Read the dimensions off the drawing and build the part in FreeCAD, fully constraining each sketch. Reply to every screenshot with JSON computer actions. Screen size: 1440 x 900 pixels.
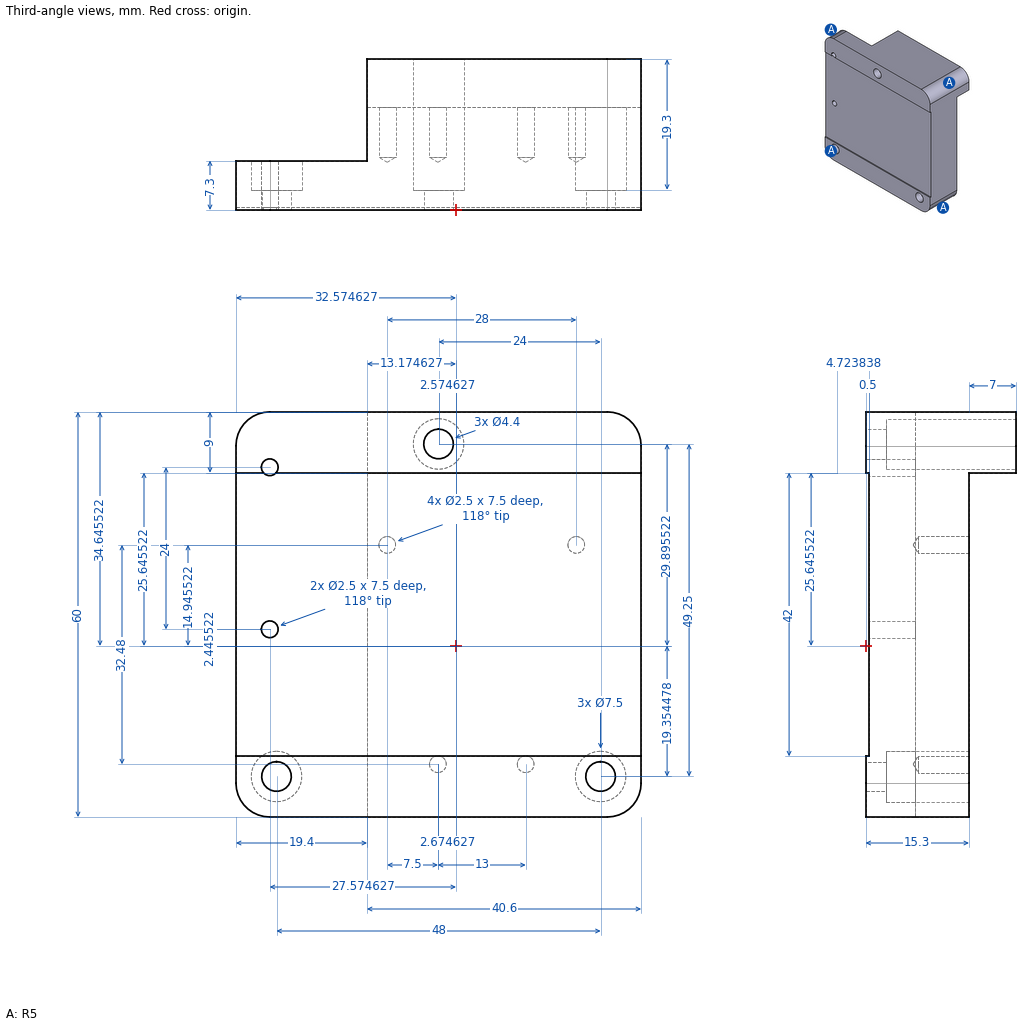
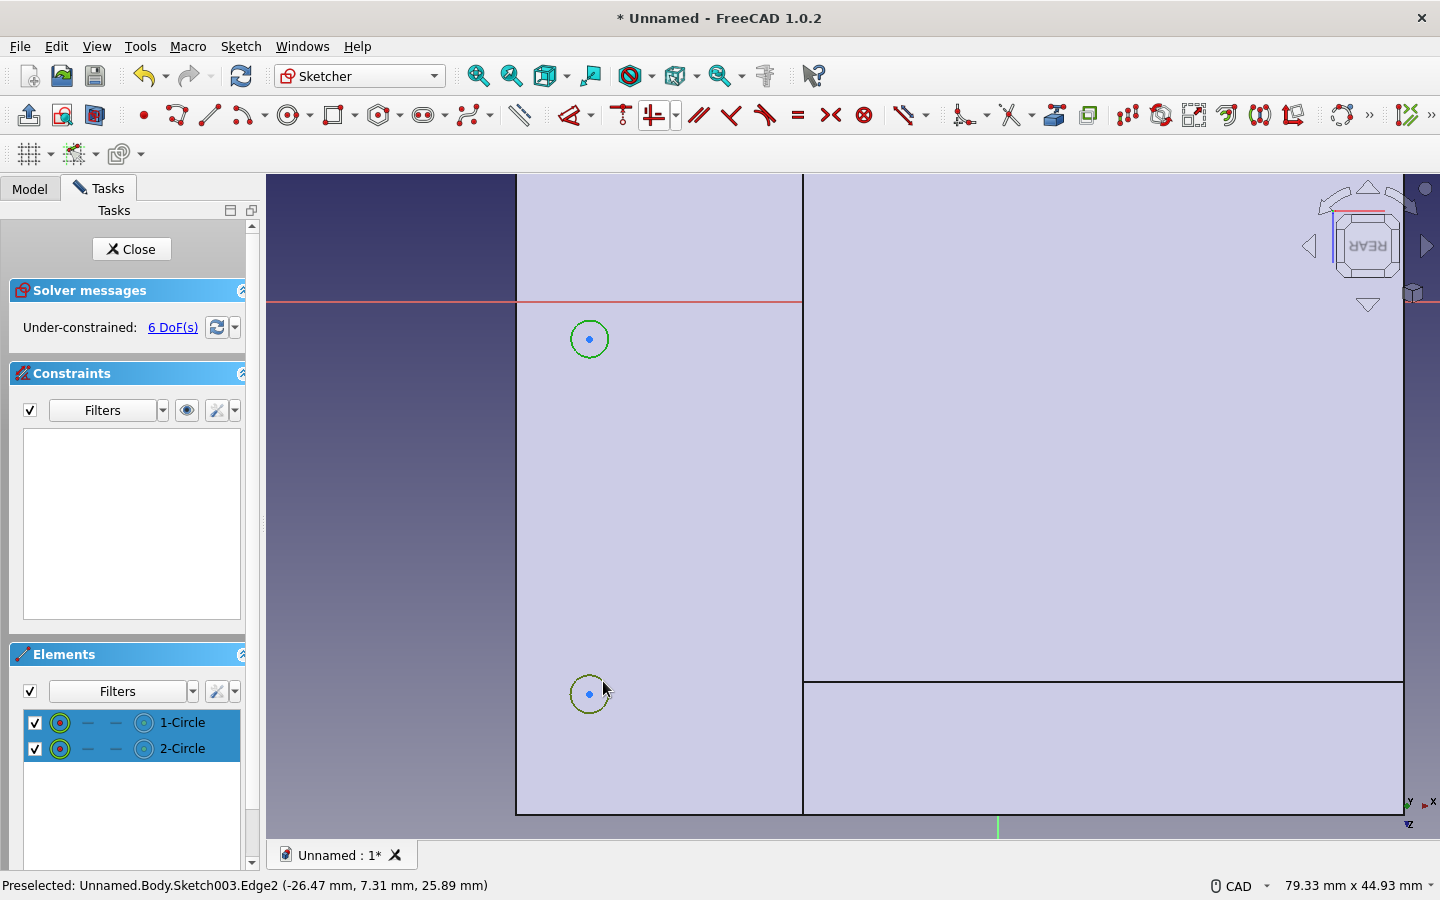
{"action": "key", "text": "e"}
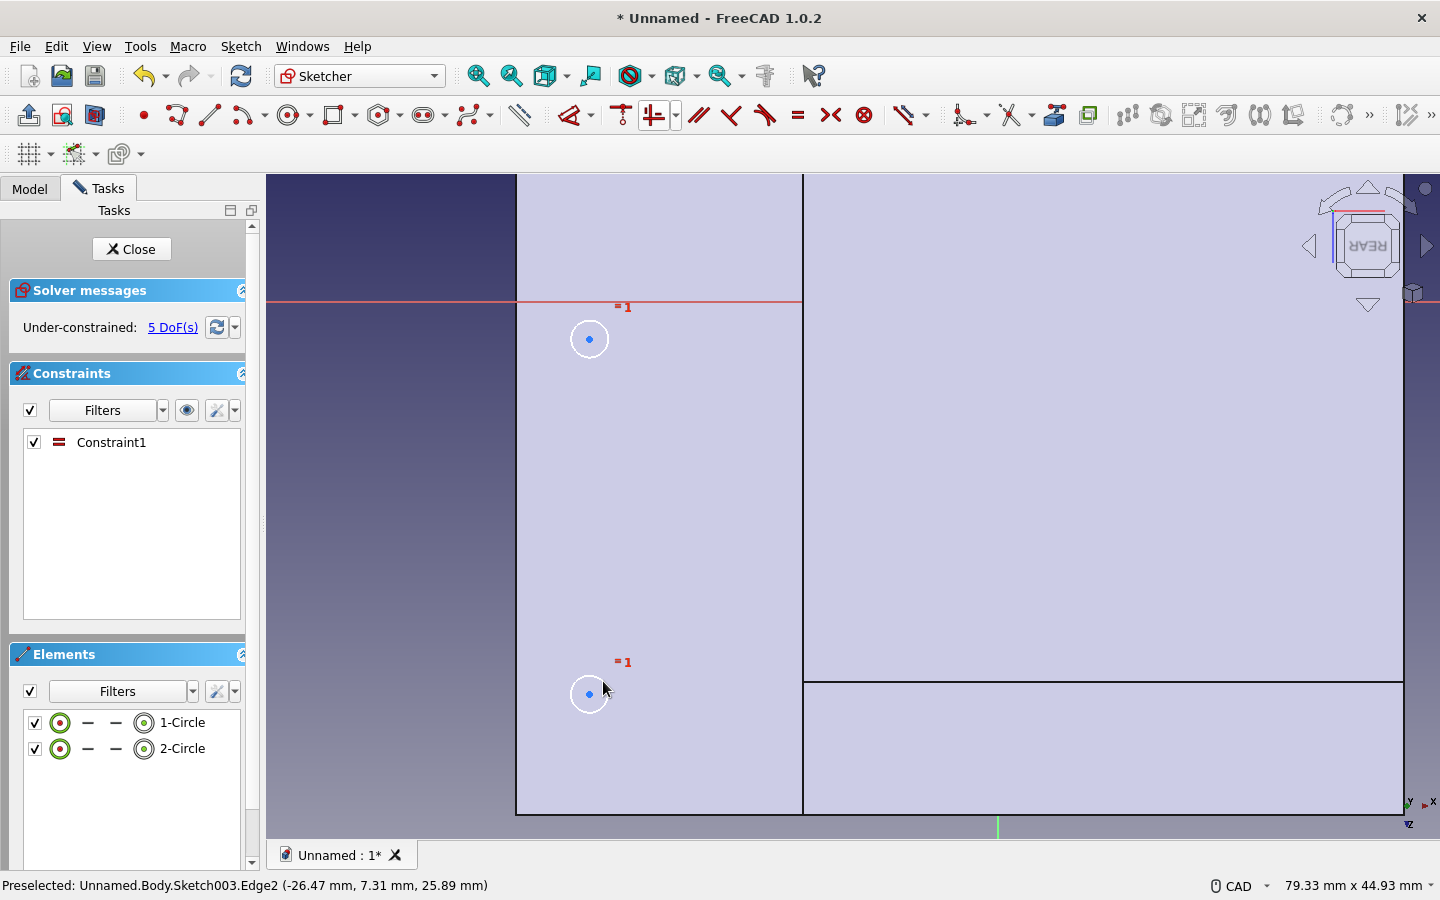
{"action": "left_click", "coordinate": [590, 339]}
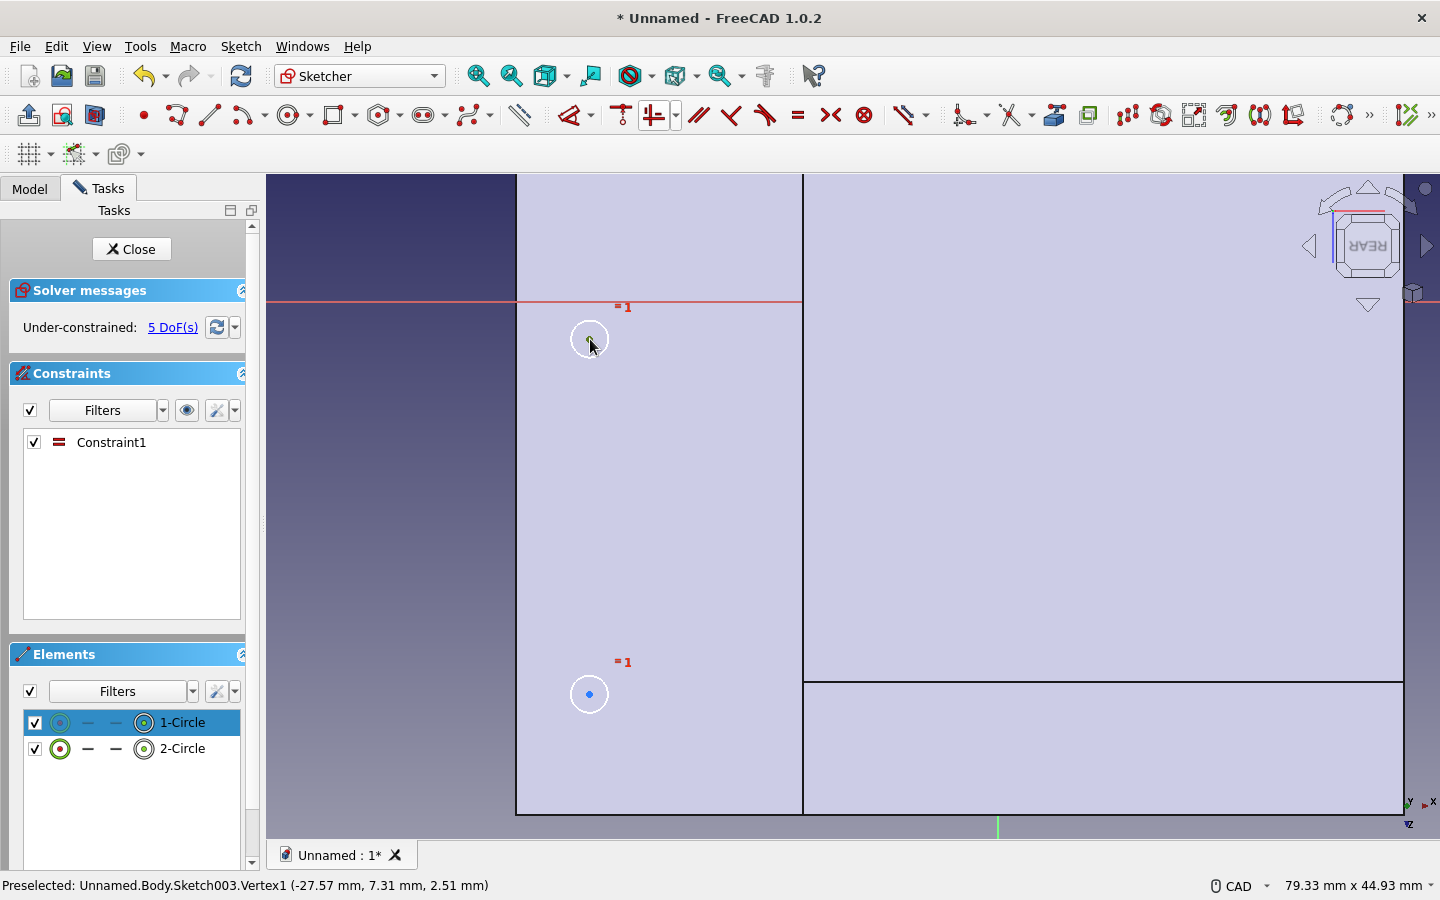
{"action": "left_click", "coordinate": [589, 694]}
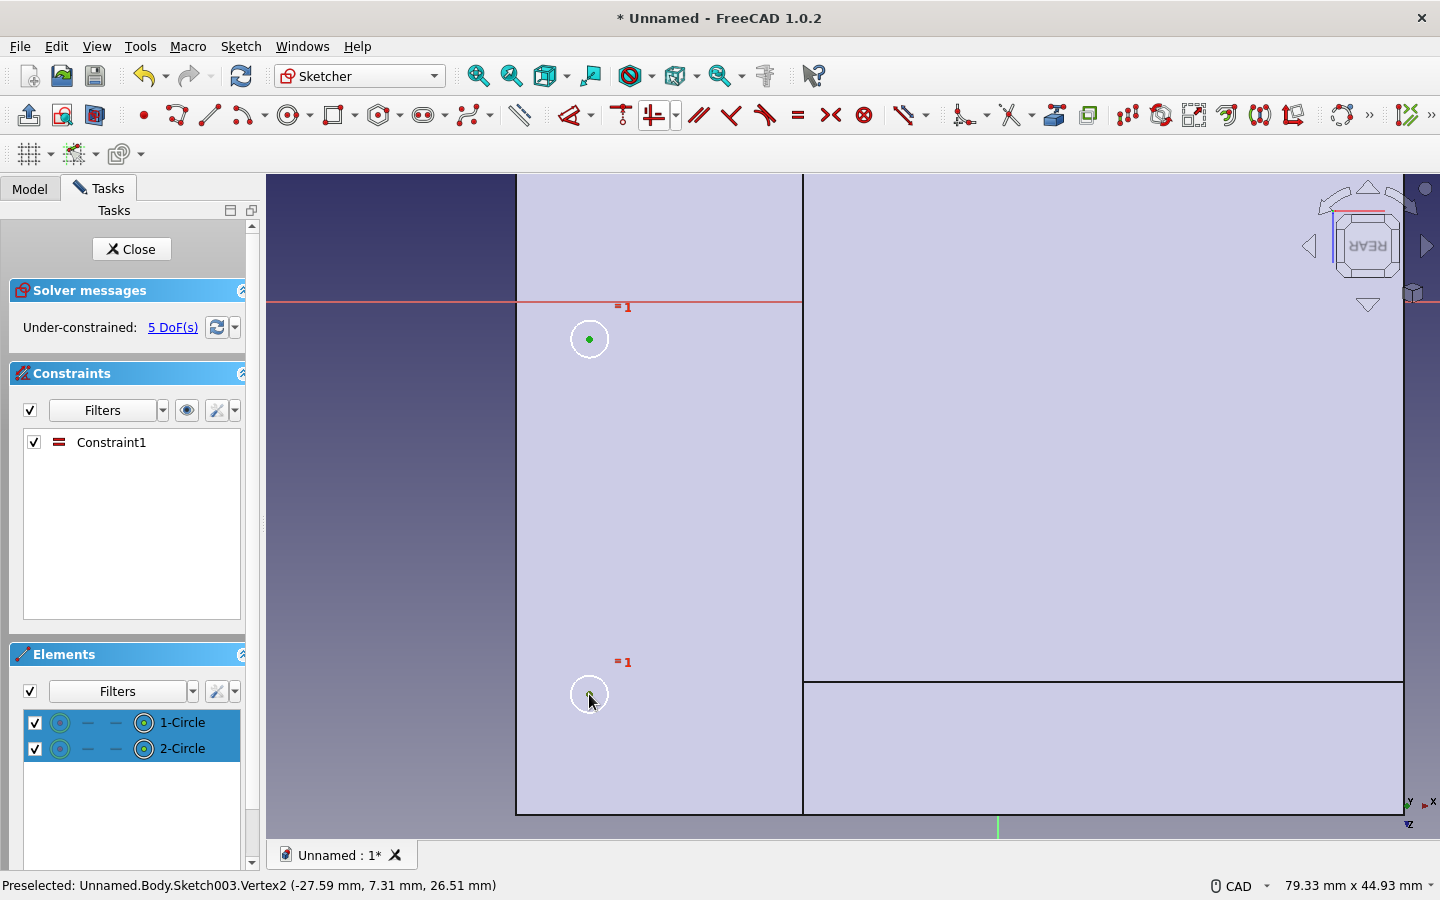
{"action": "key", "text": "v"}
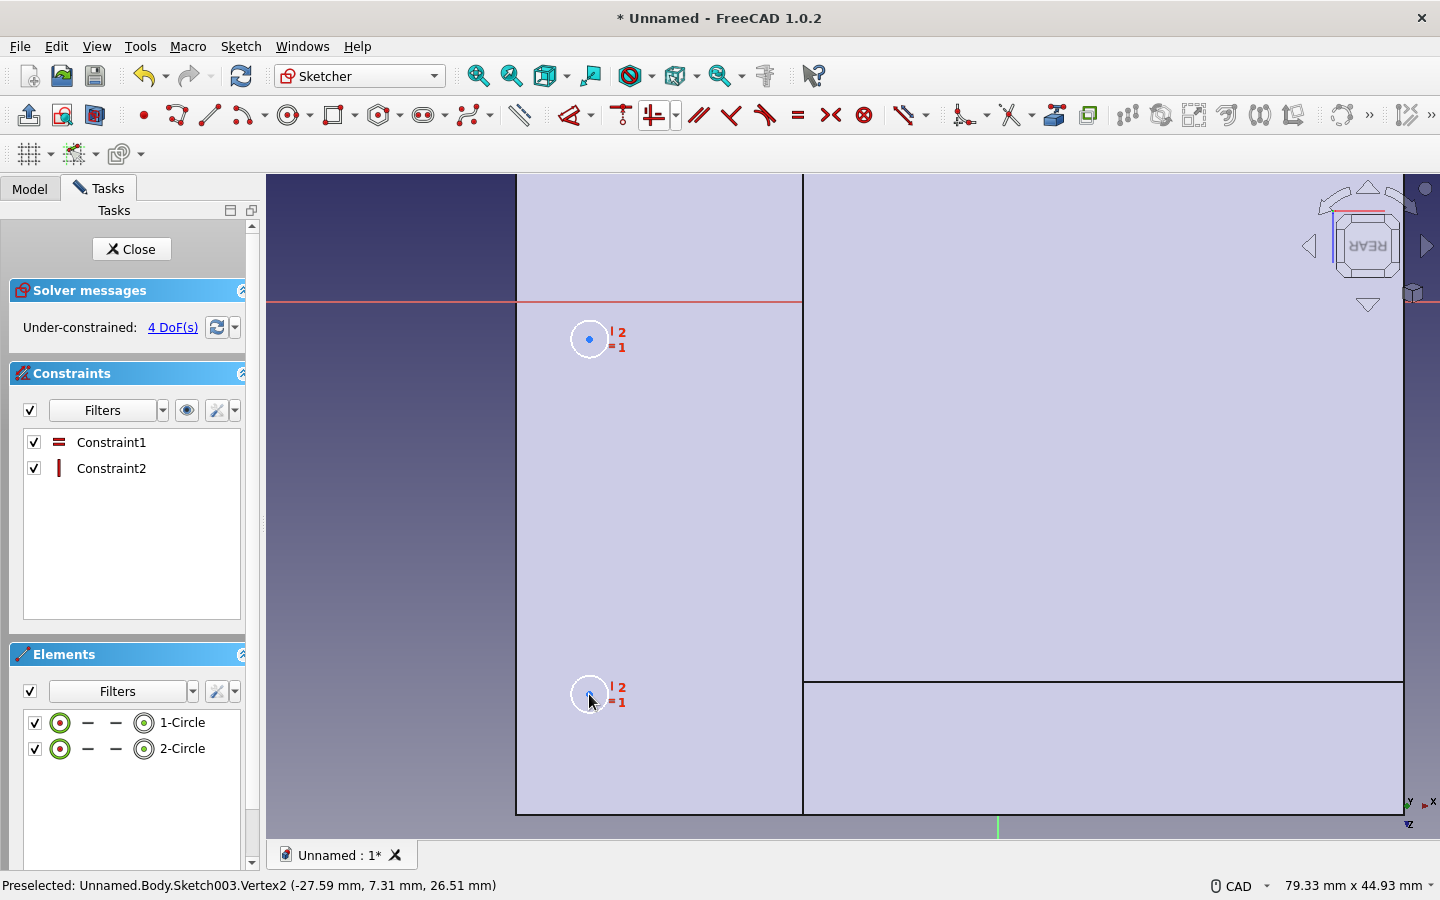
{"action": "key", "text": "d"}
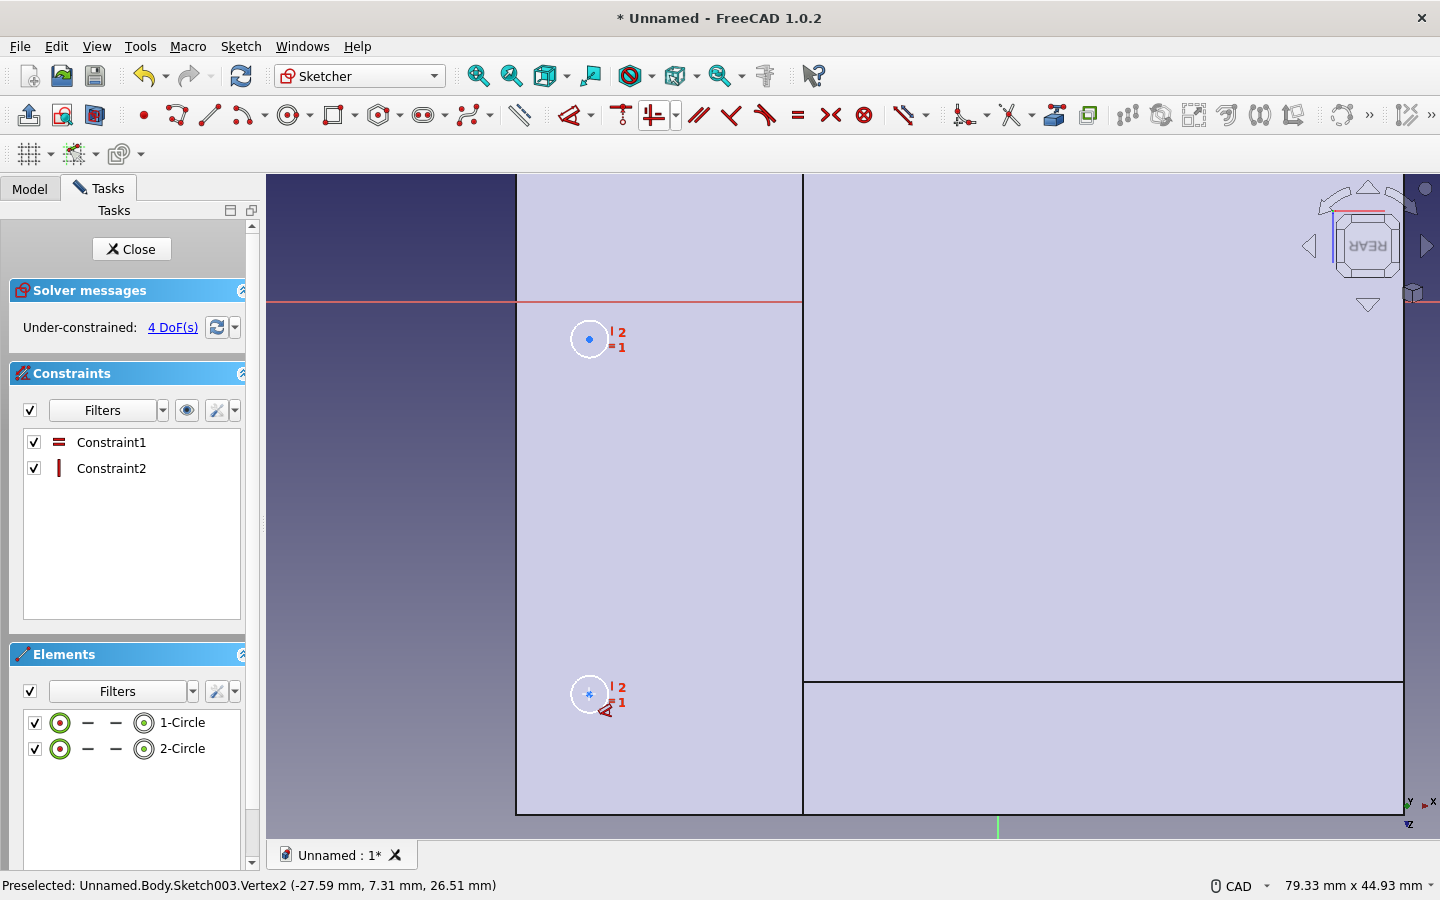
{"action": "left_click", "coordinate": [603, 326]}
{"action": "left_click", "coordinate": [638, 325]}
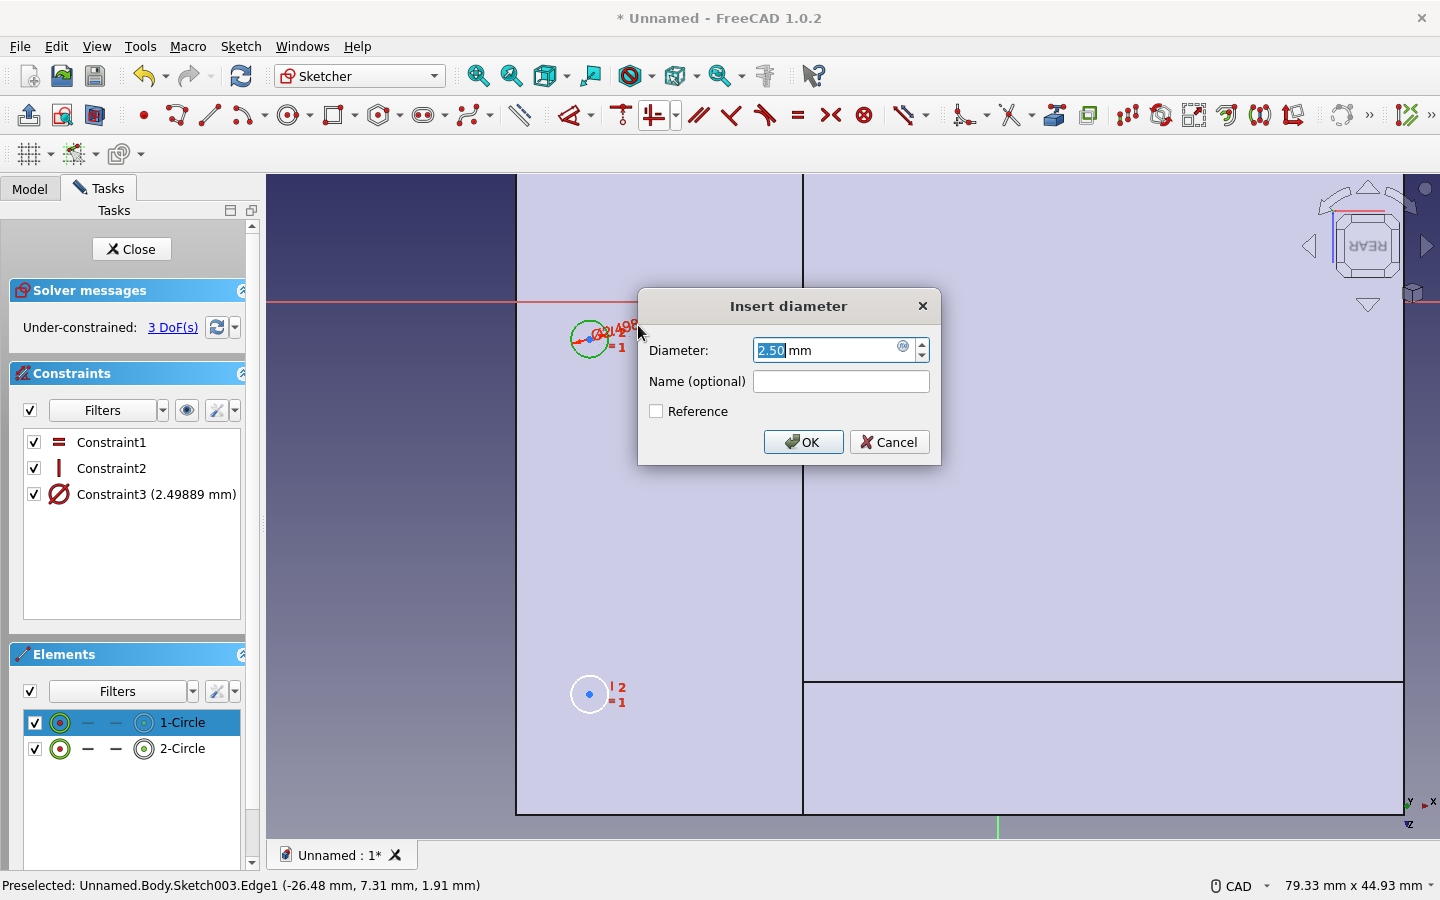
{"action": "type", "text": "2.5"}
{"action": "key", "text": "Return"}